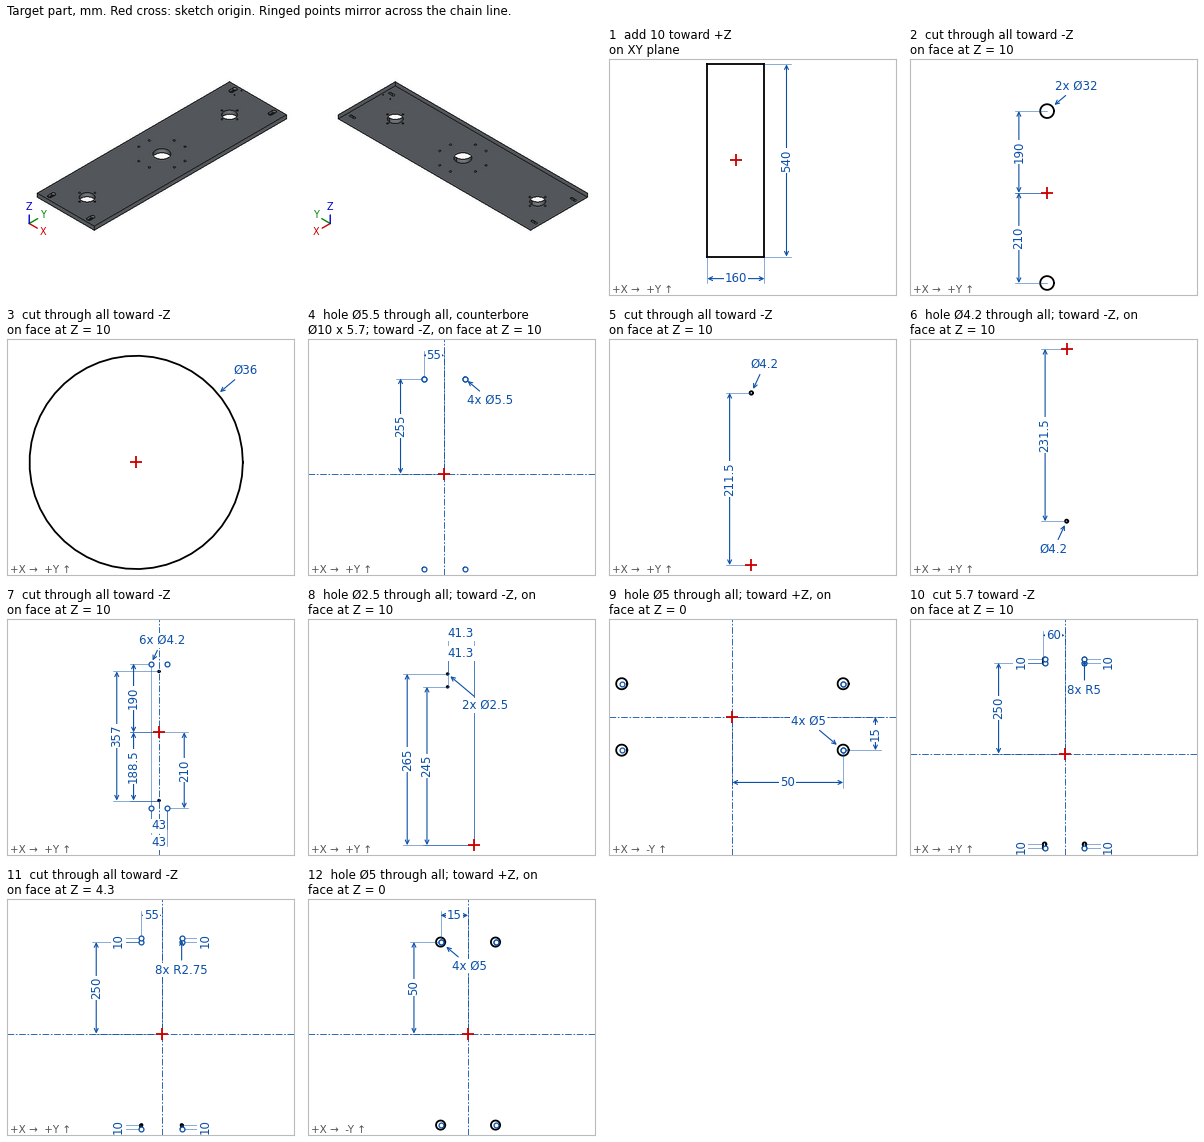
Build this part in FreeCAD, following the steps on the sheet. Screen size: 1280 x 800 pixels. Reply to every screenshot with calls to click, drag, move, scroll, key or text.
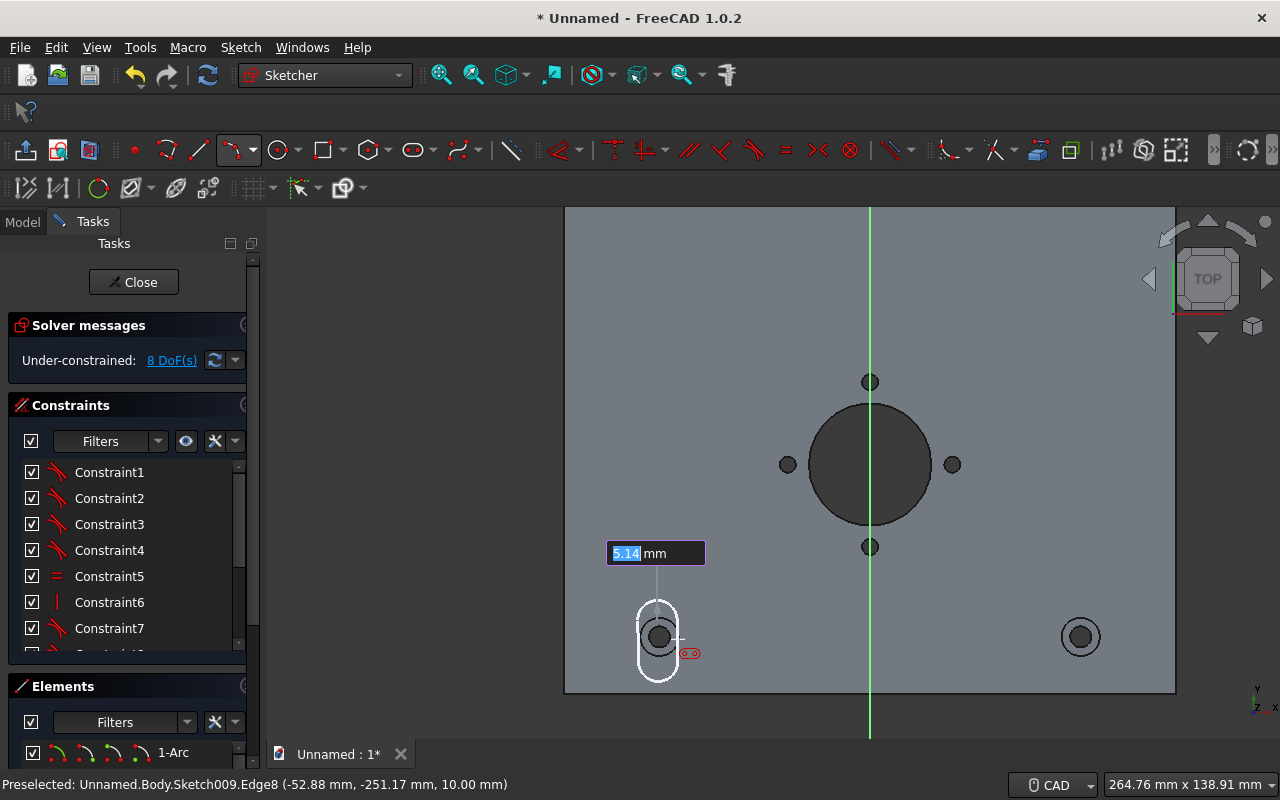
click(679, 637)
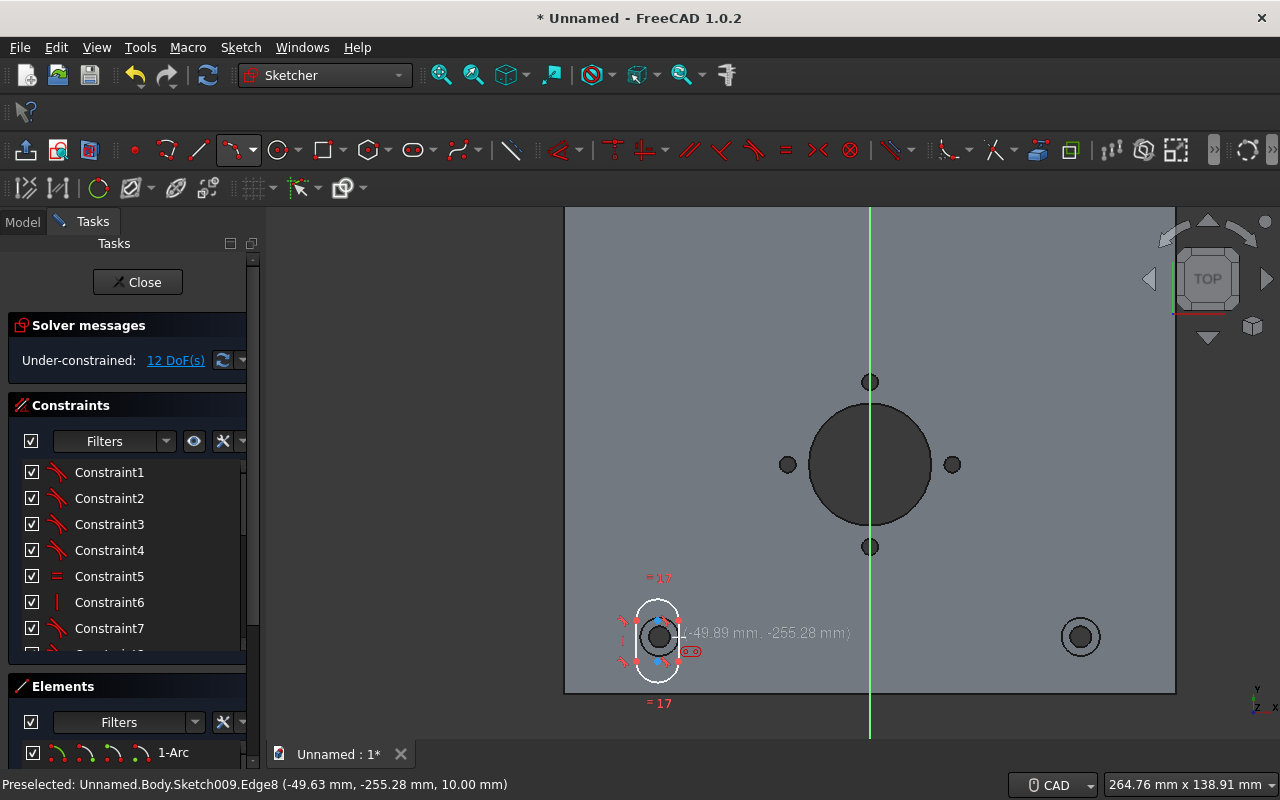
scroll(672, 634, down, 9)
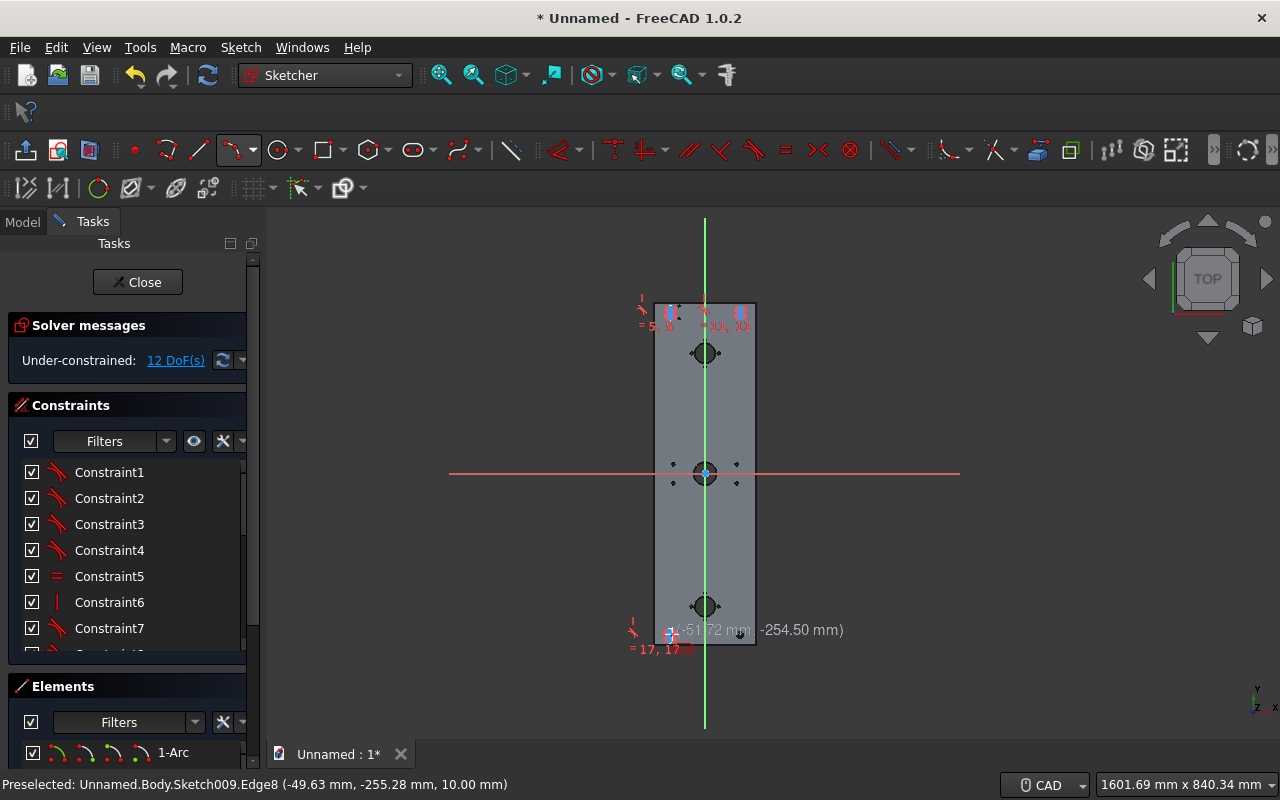
click(740, 638)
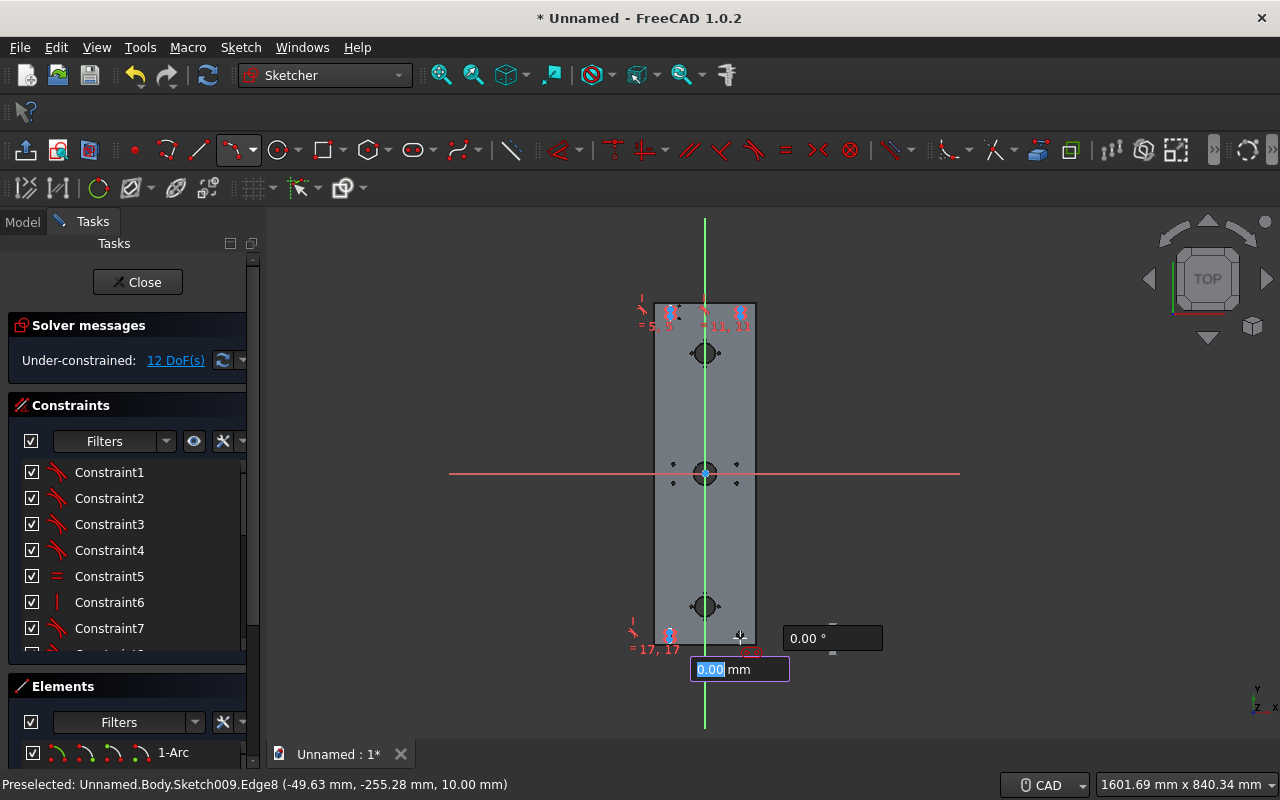
scroll(740, 632, up, 5)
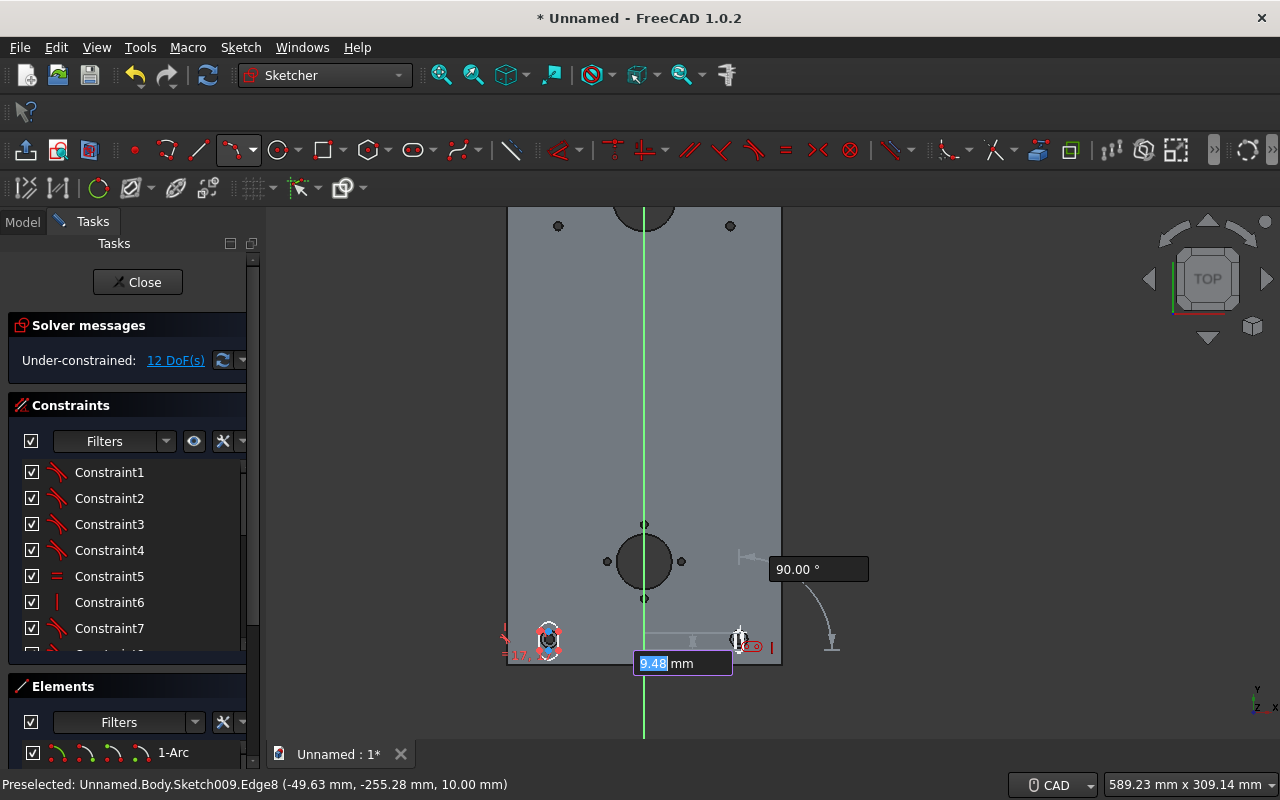
click(739, 631)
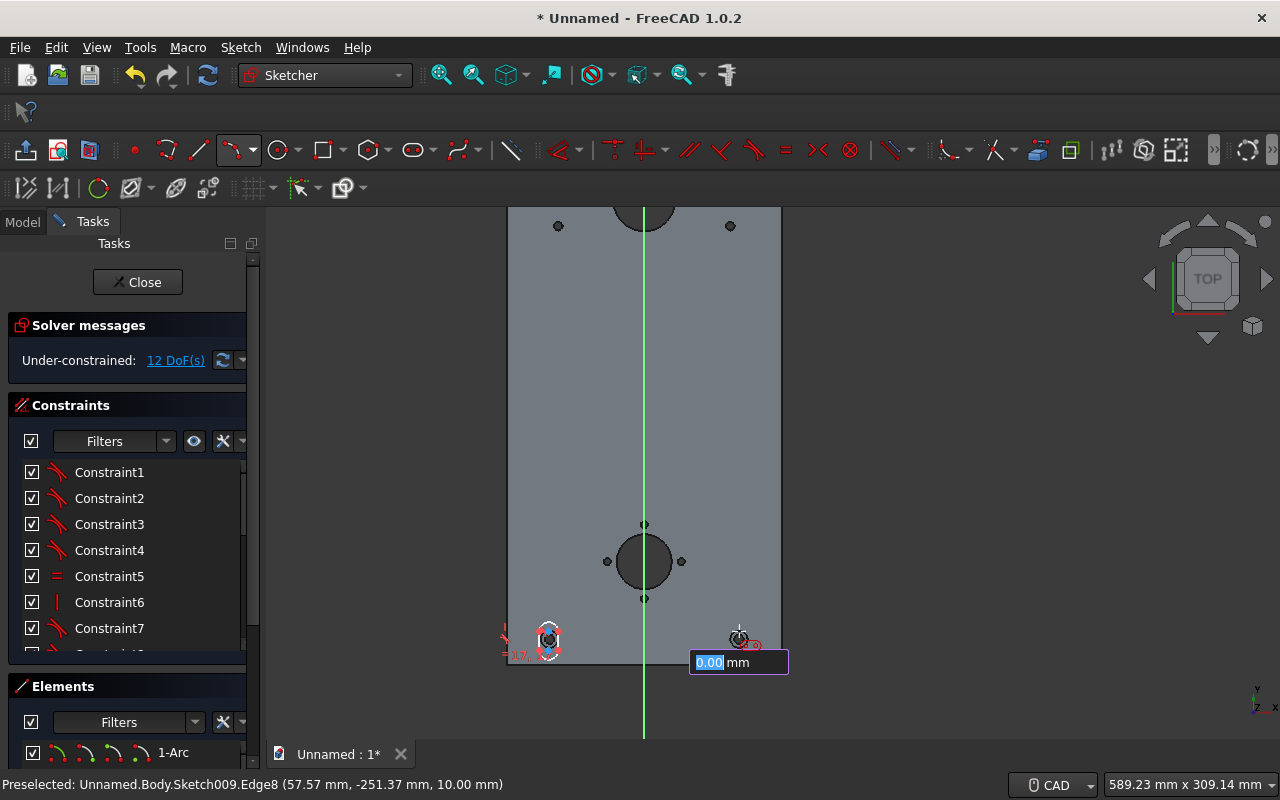
scroll(748, 639, up, 4)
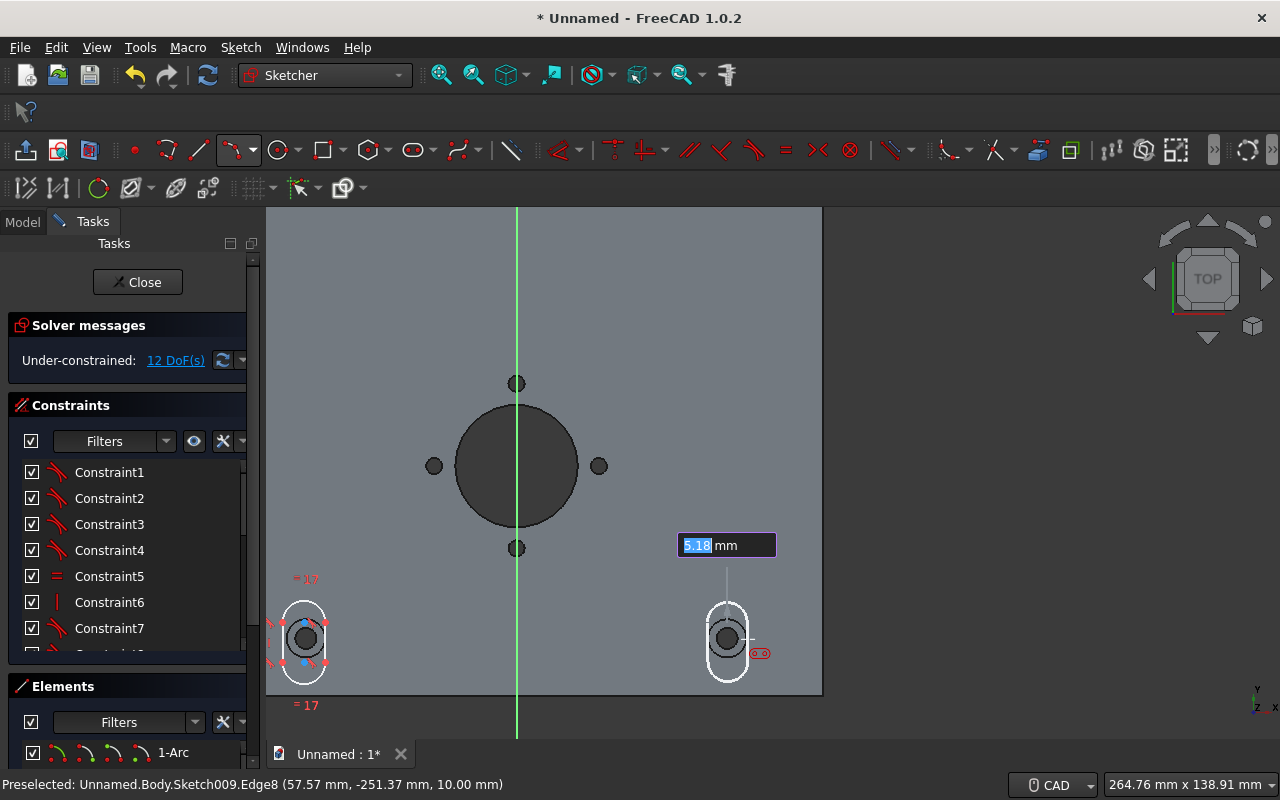
click(746, 638)
key(Escape)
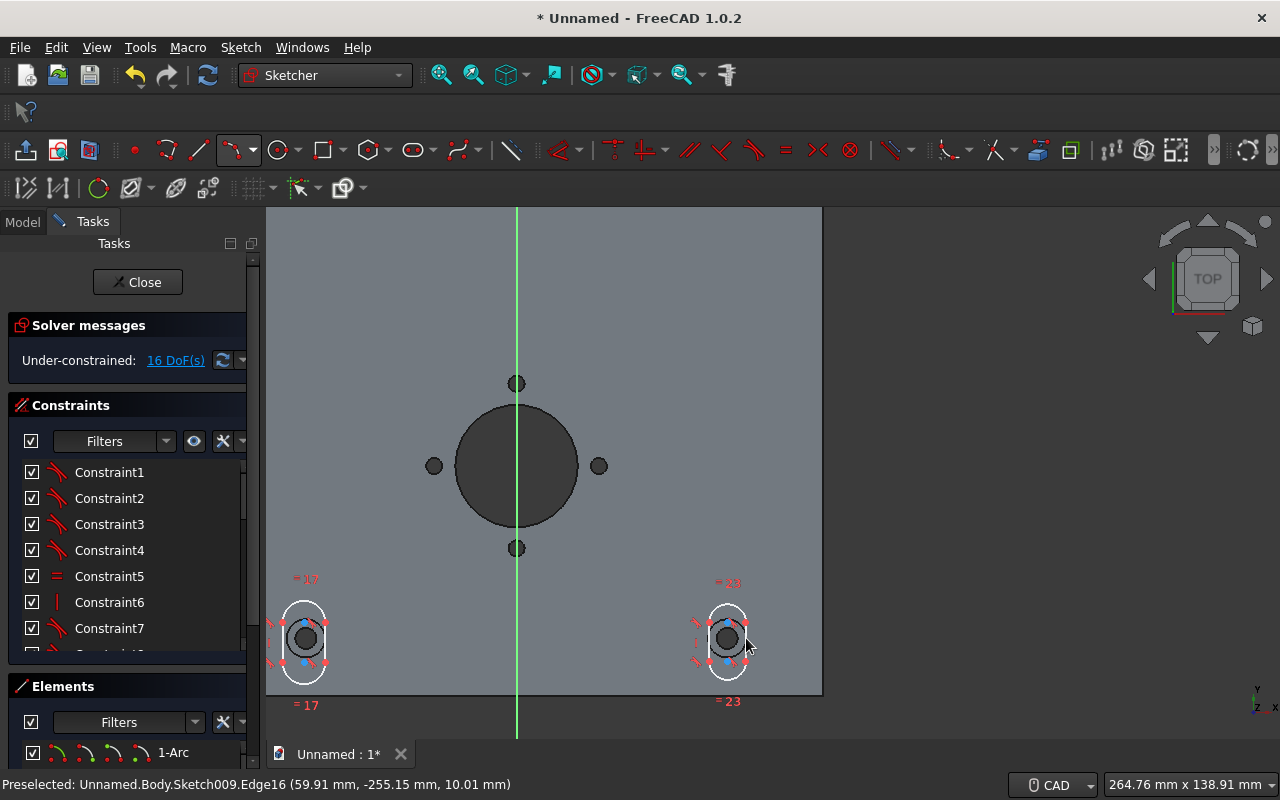
scroll(742, 634, down, 9)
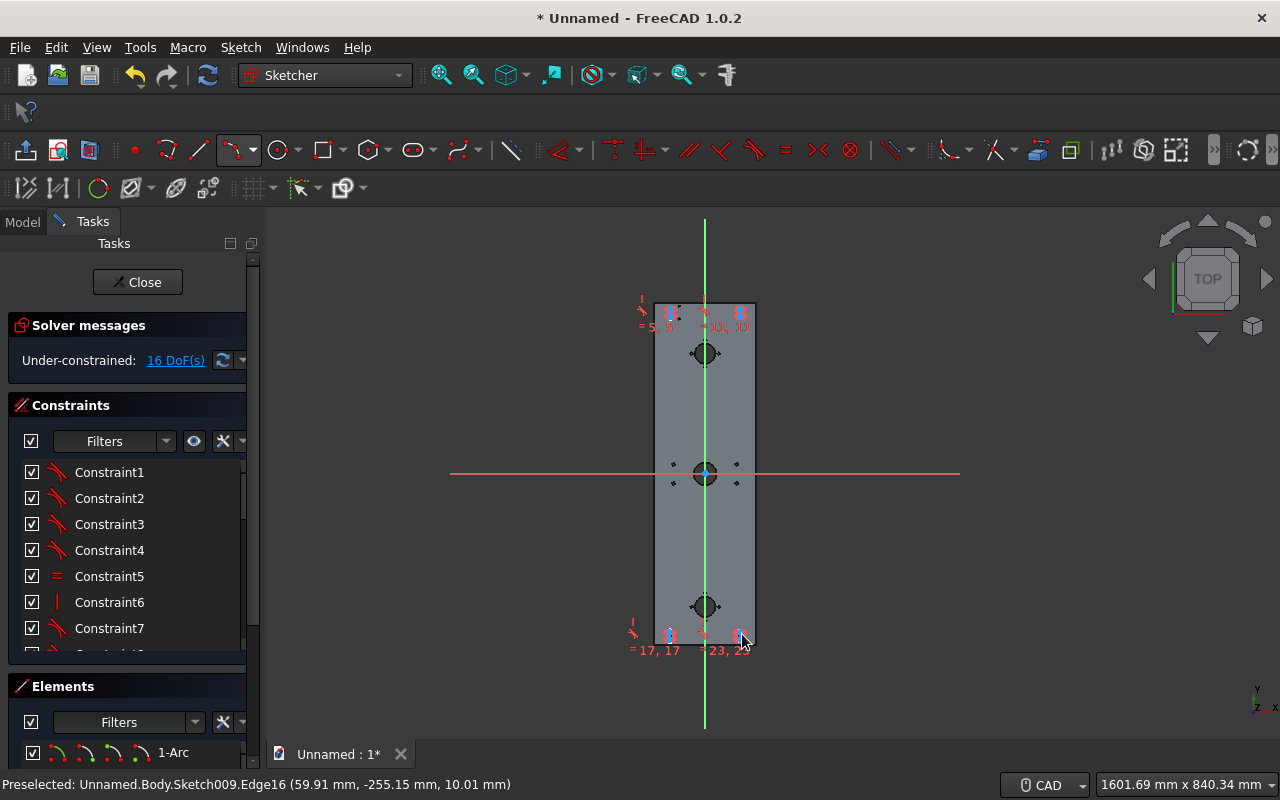
scroll(669, 319, up, 9)